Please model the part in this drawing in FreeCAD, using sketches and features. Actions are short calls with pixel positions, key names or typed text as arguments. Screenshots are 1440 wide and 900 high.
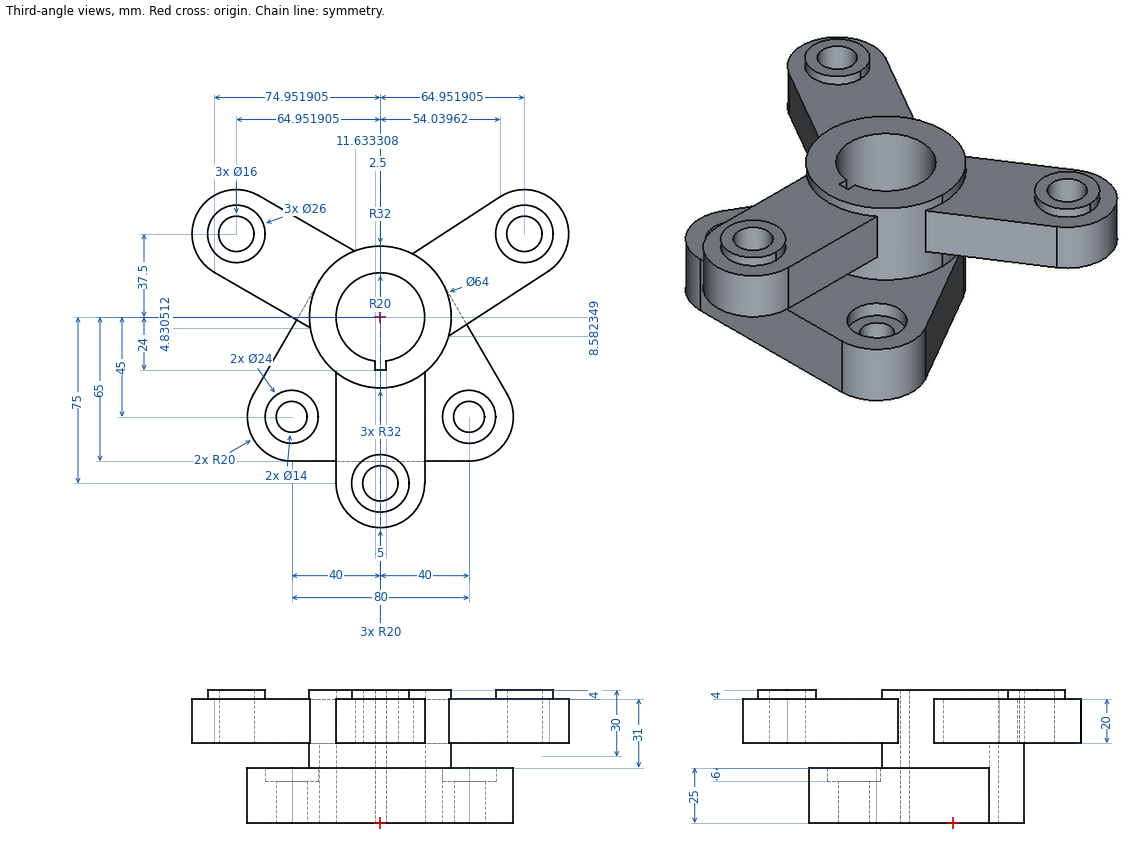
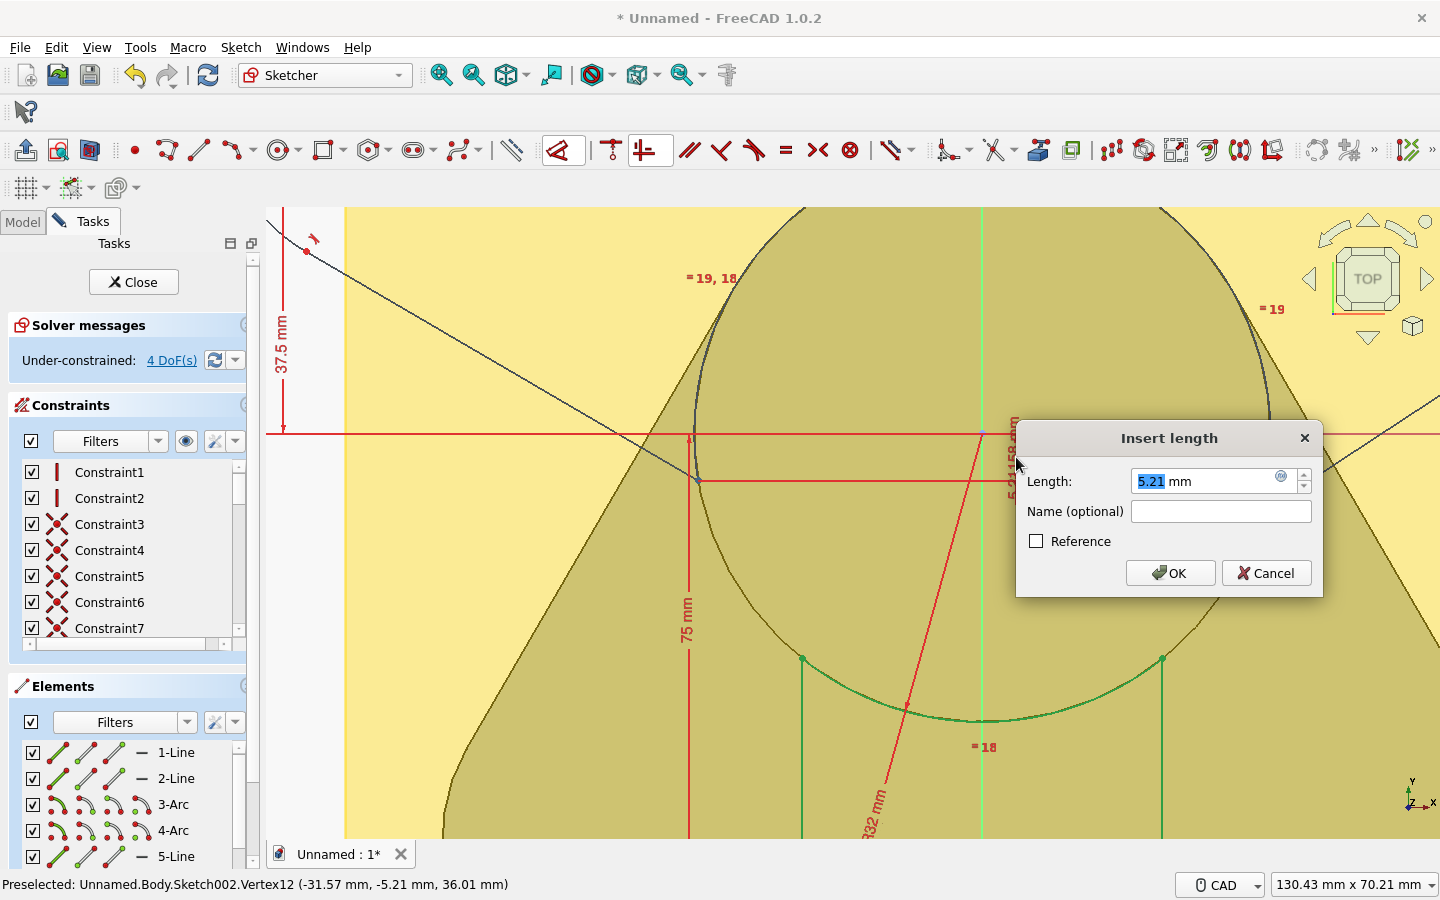
text(4.830512)
key(Return)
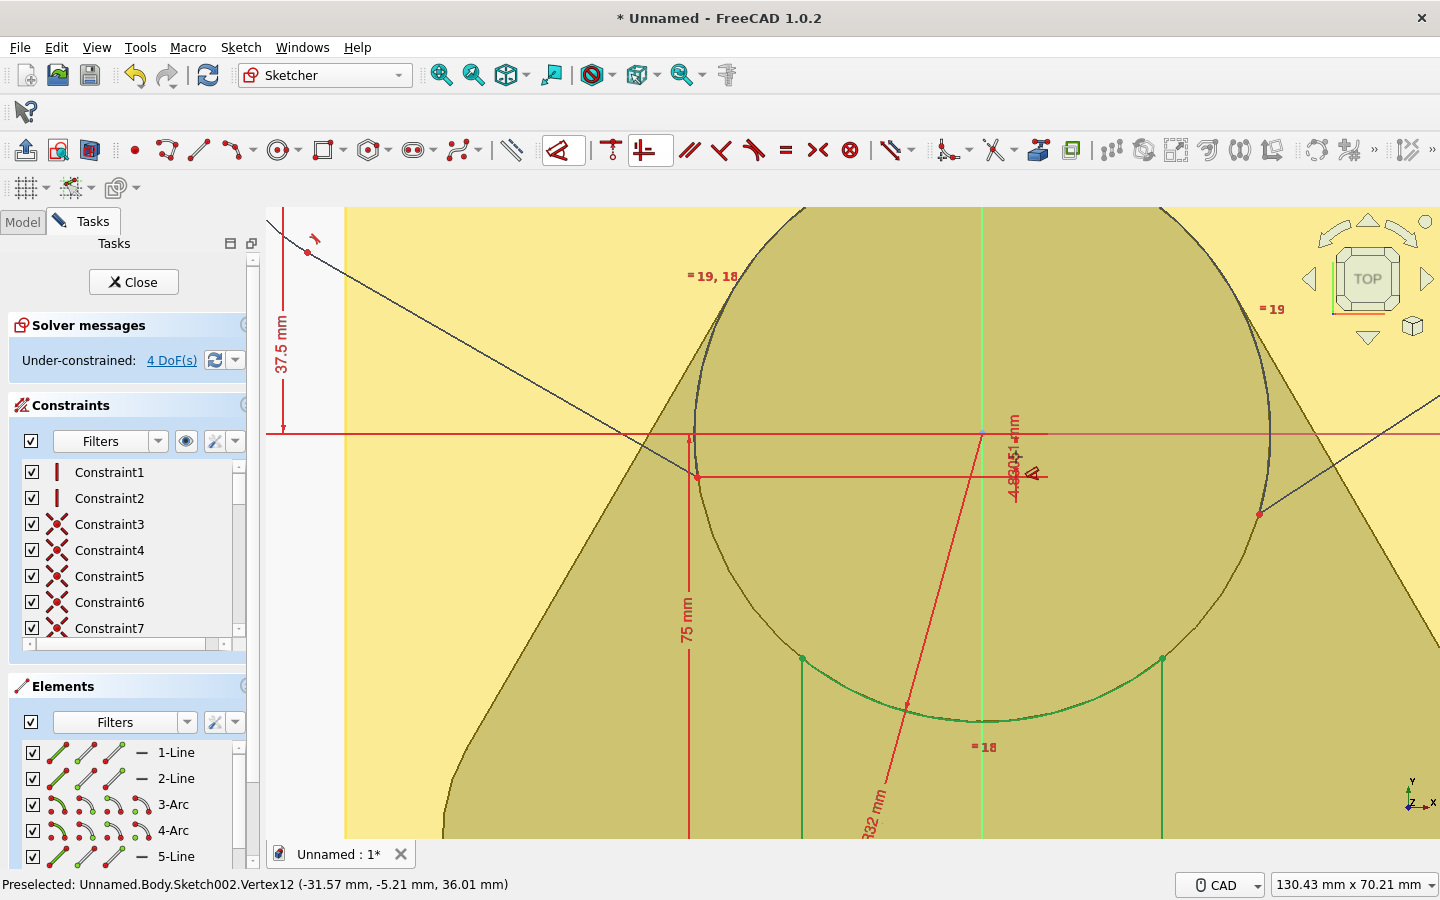
scroll(700, 483, down, 6)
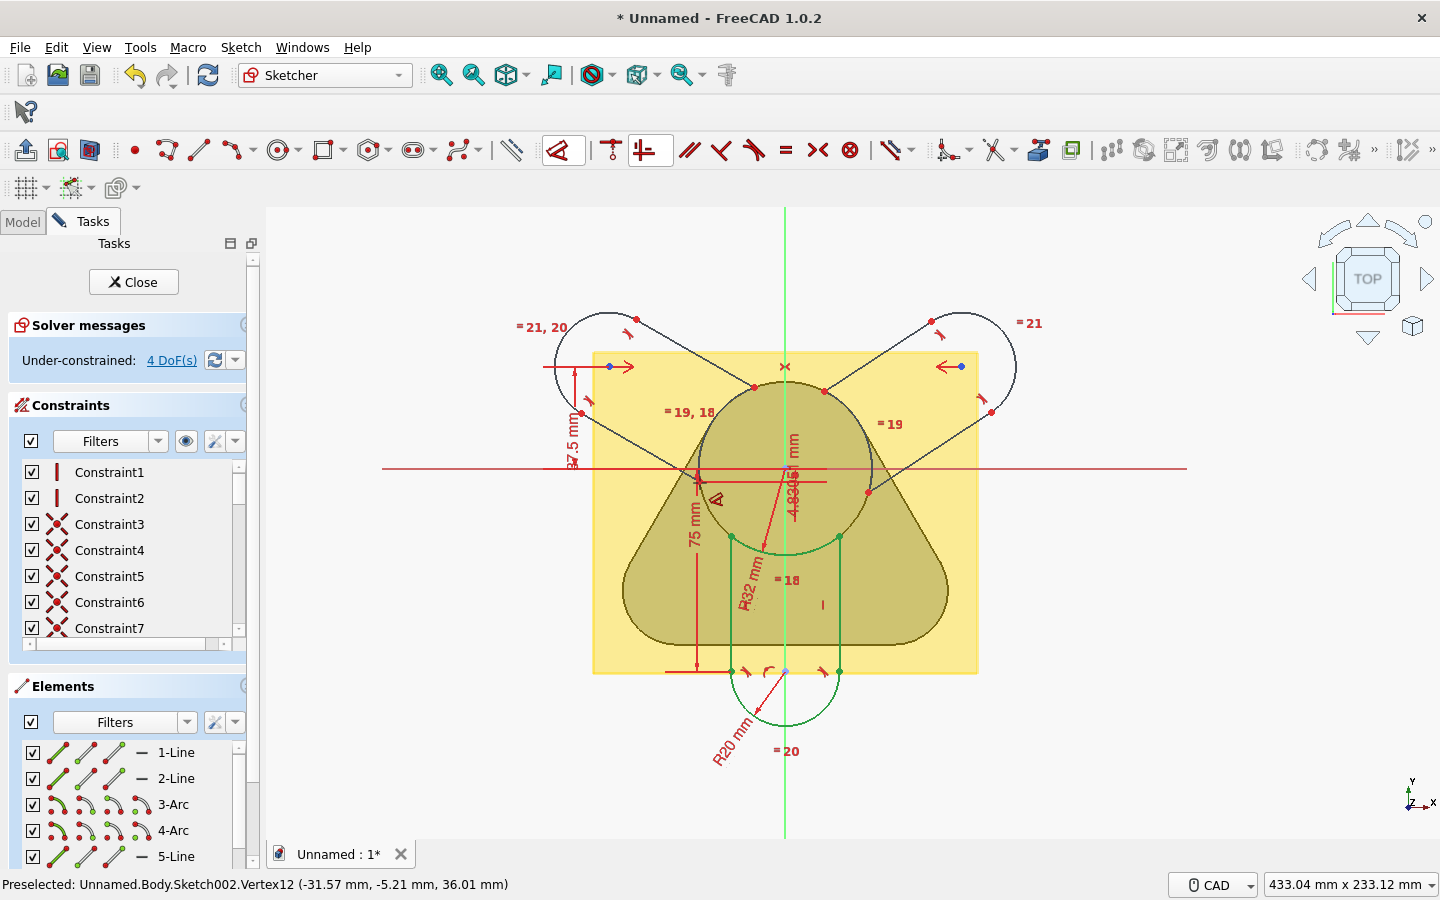
click(932, 321)
click(859, 287)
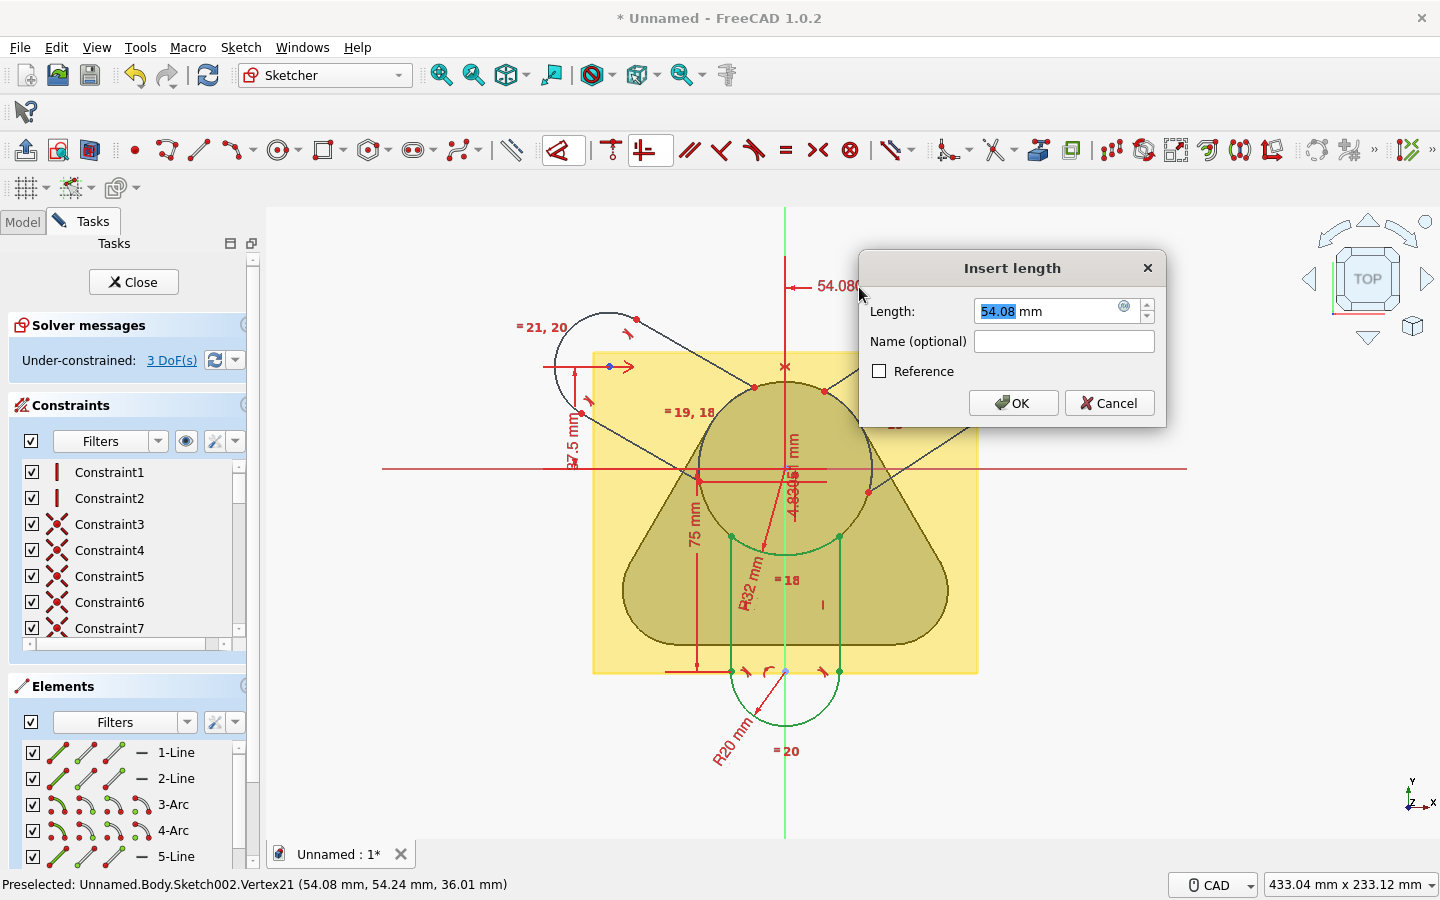
text(54.03962)
key(Return)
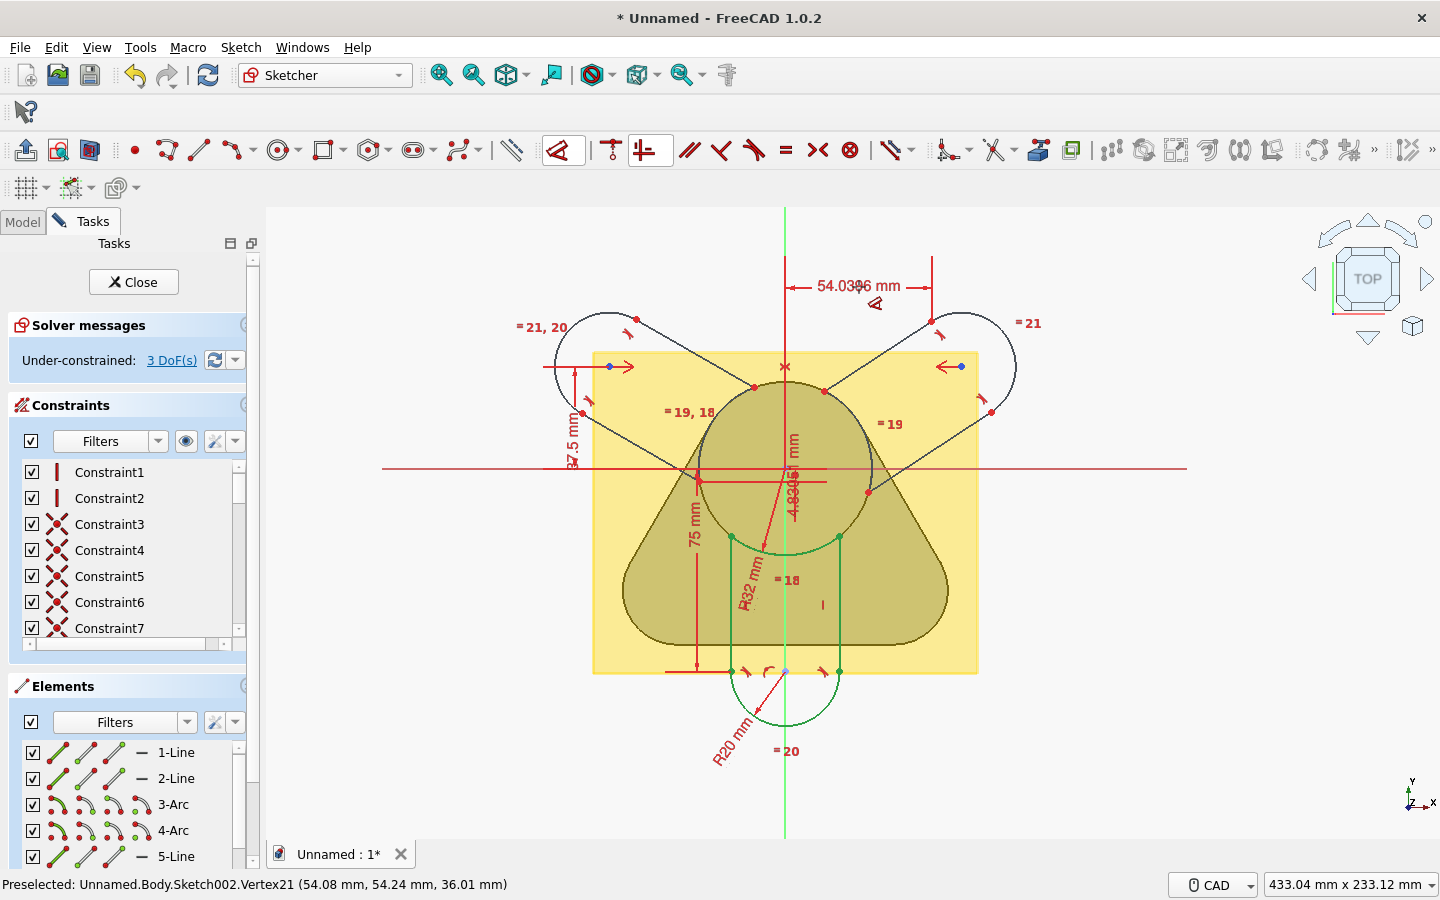
scroll(869, 493, up, 3)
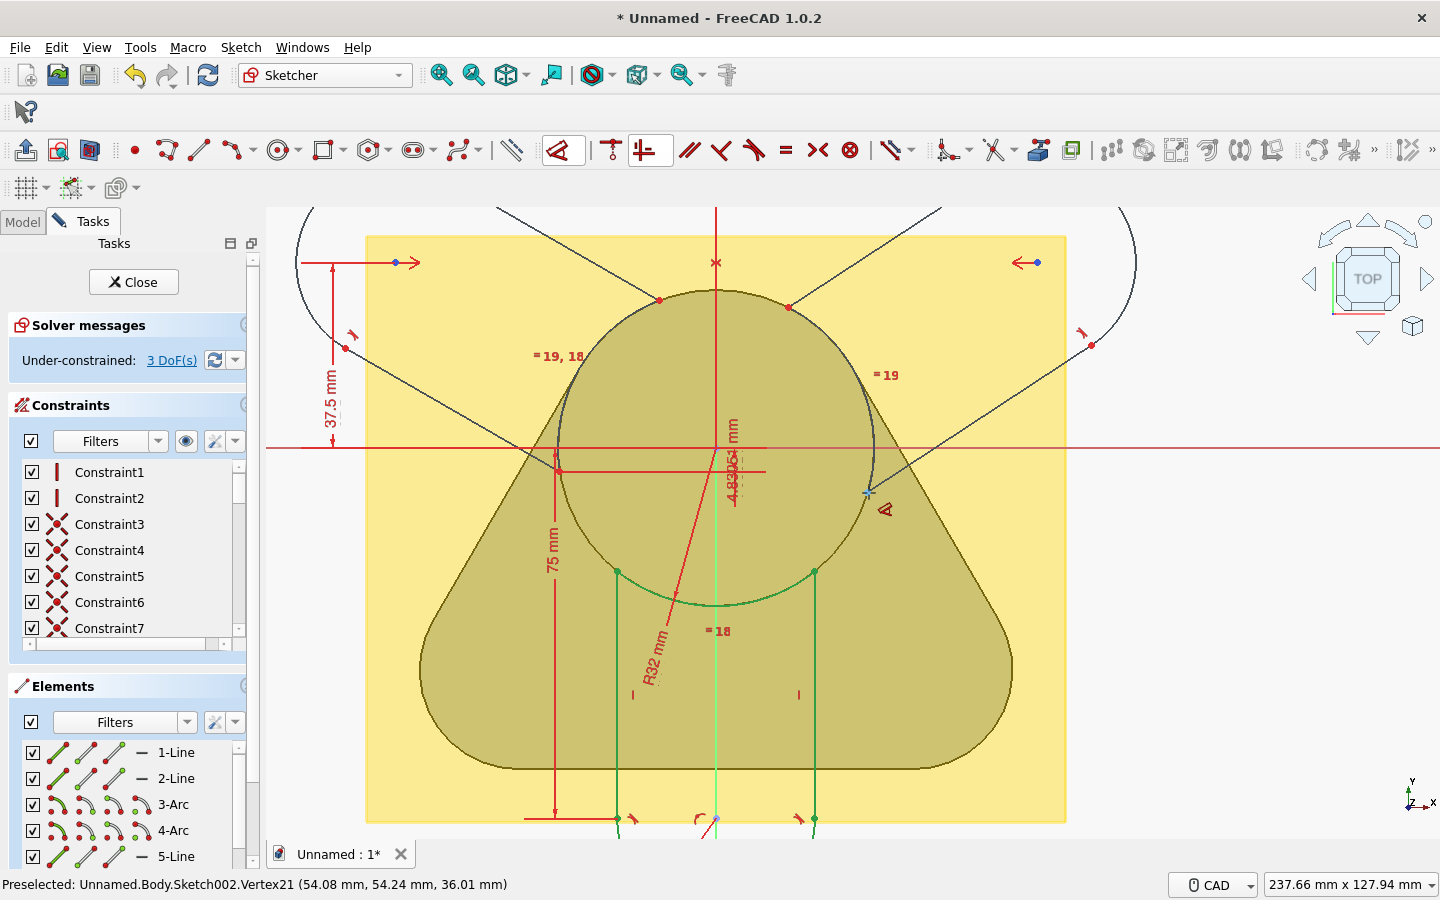
click(868, 492)
click(902, 485)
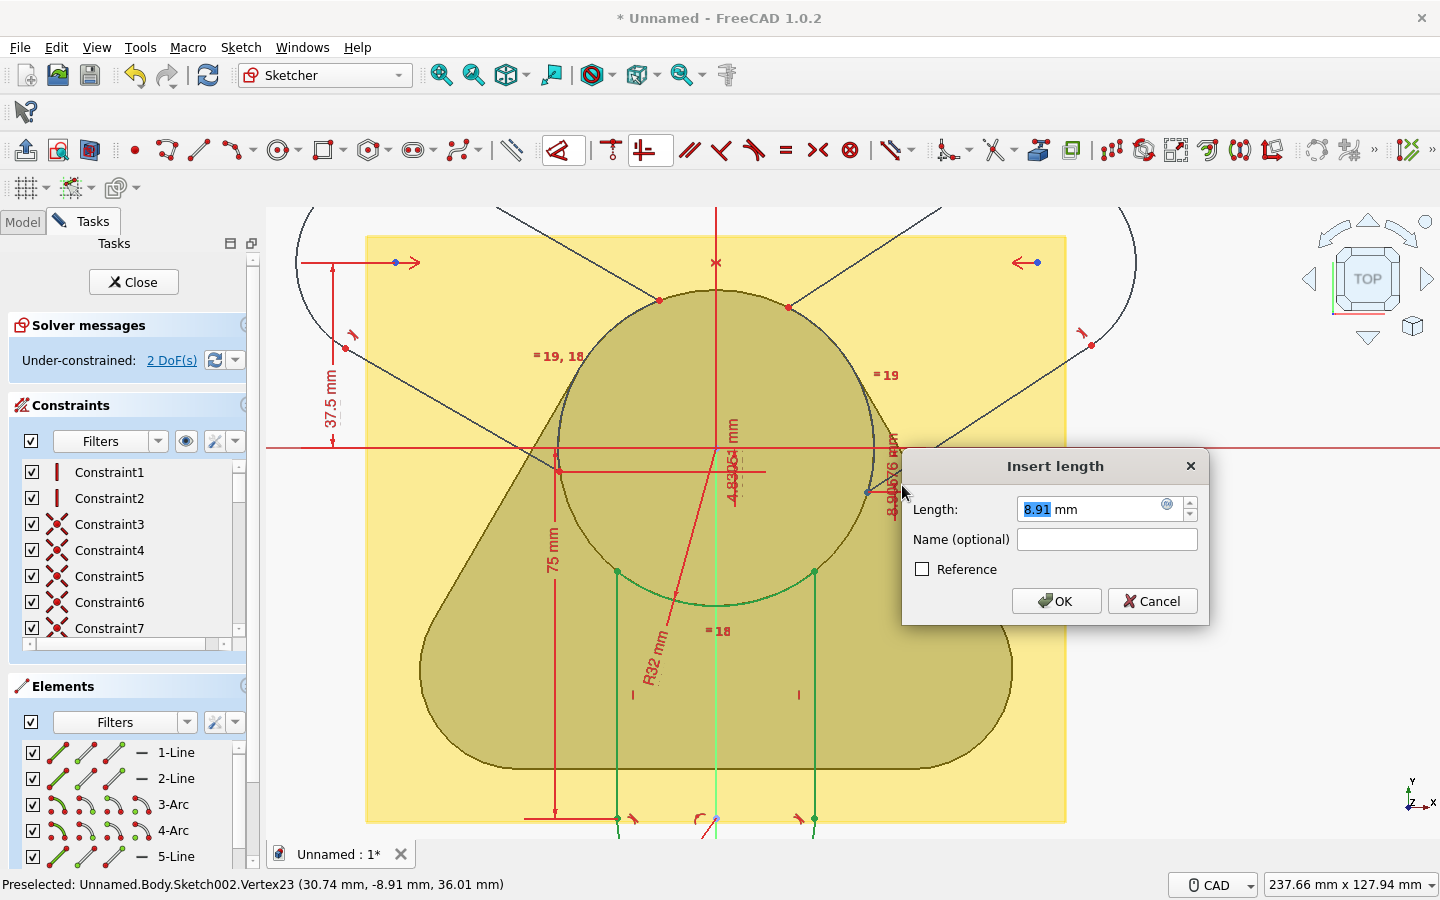
text(8.582349)
key(Return)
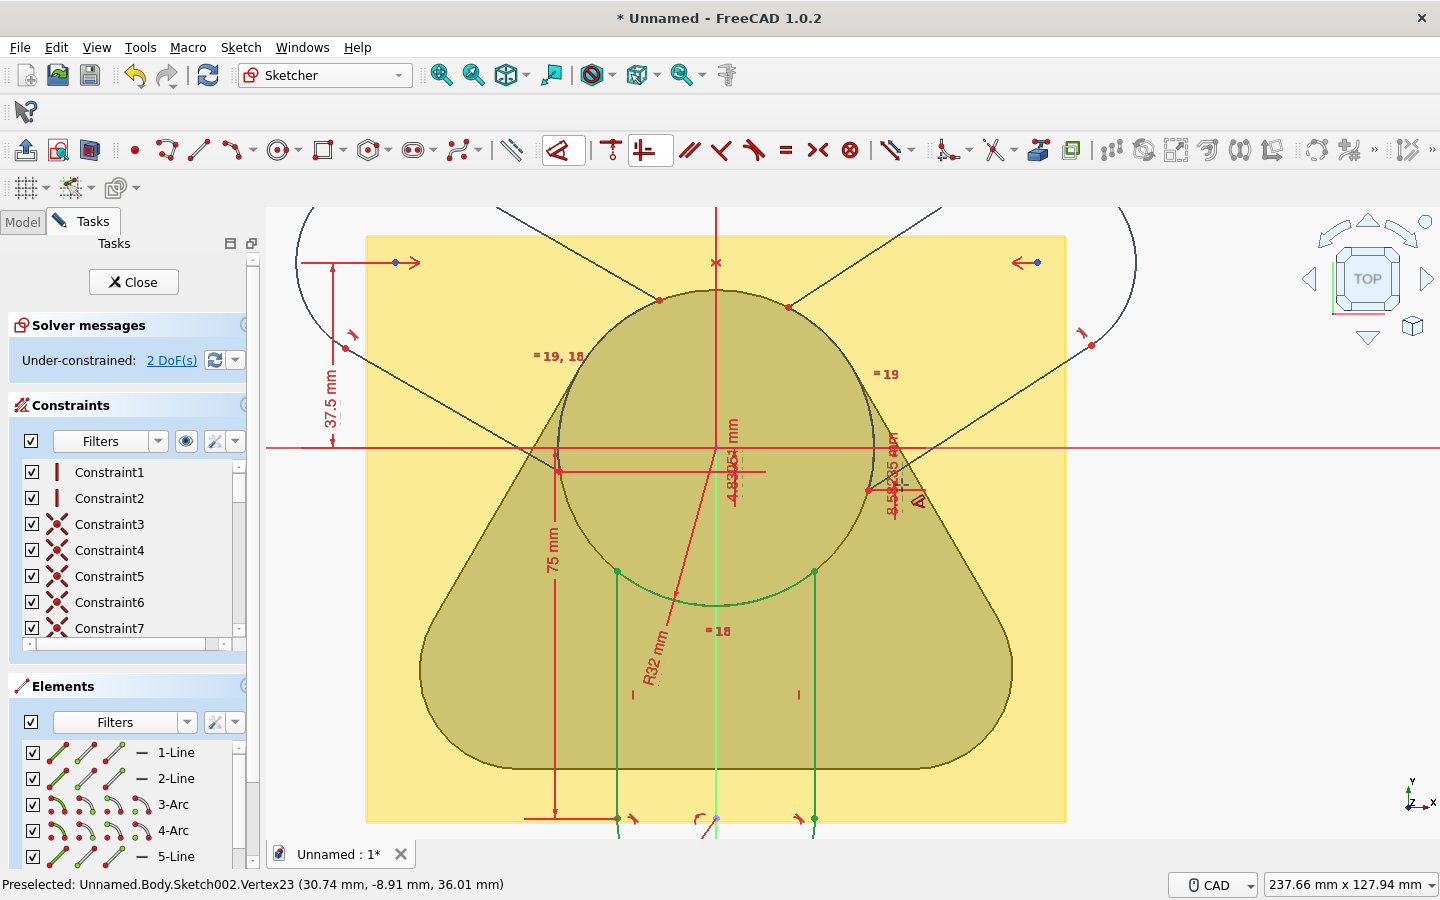
click(346, 348)
click(531, 314)